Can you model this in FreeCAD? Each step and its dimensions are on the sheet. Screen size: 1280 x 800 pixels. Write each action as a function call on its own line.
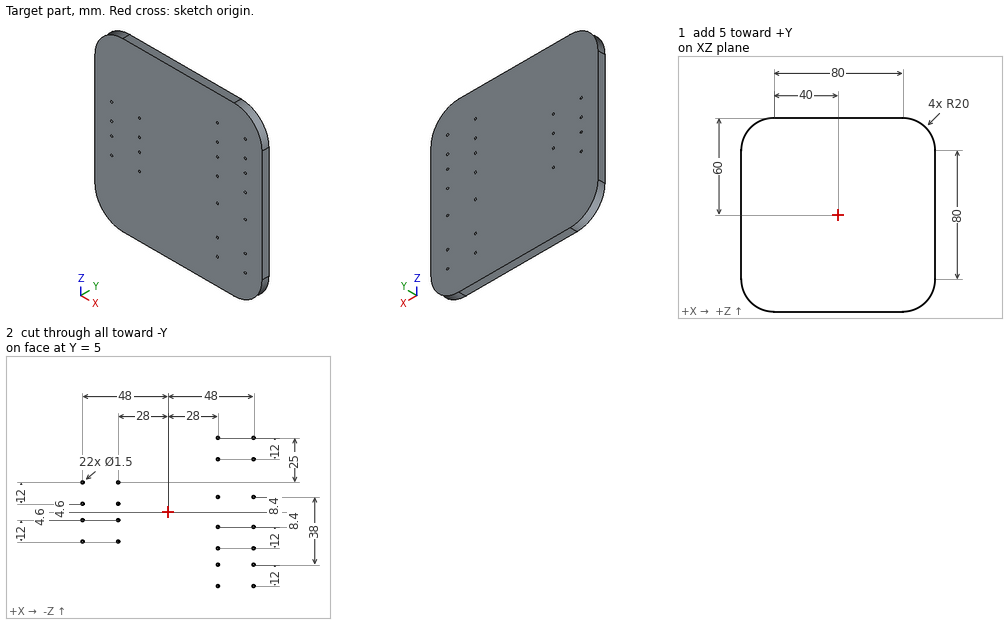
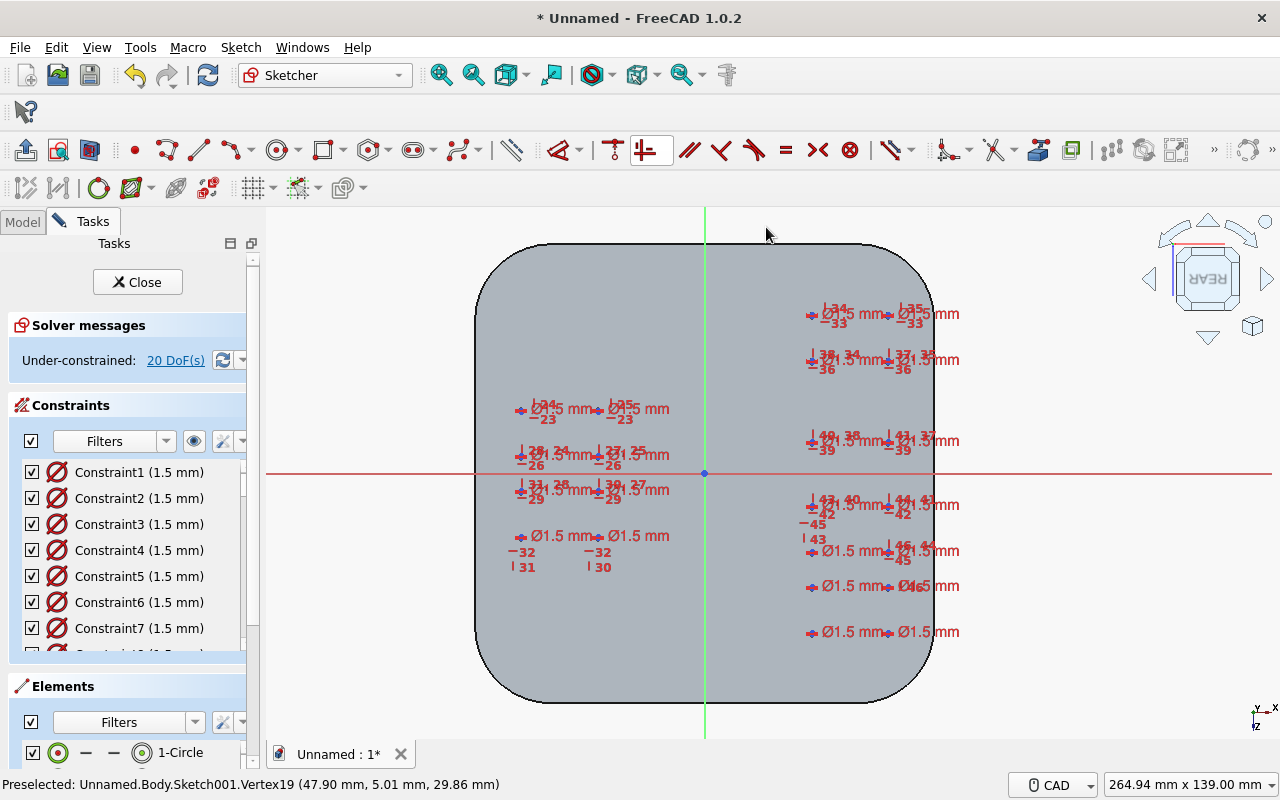
click(812, 553)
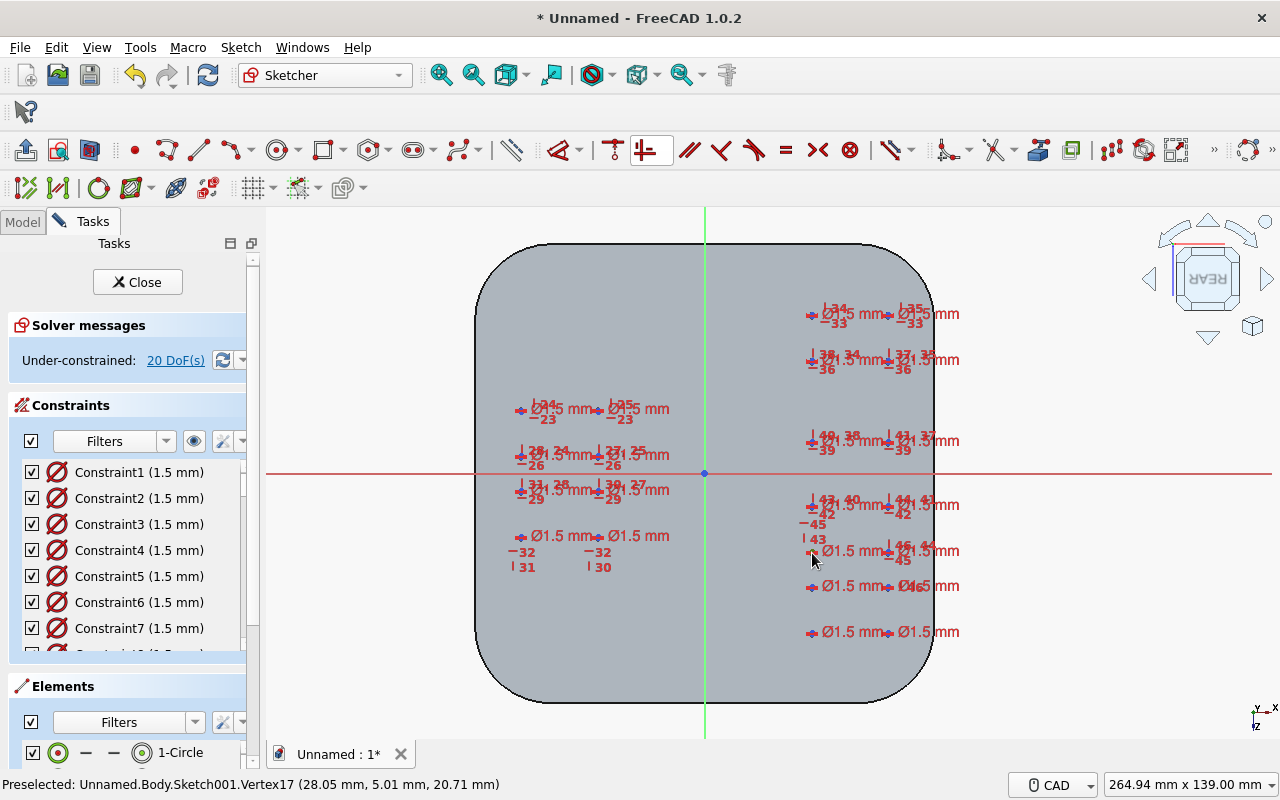
click(812, 588)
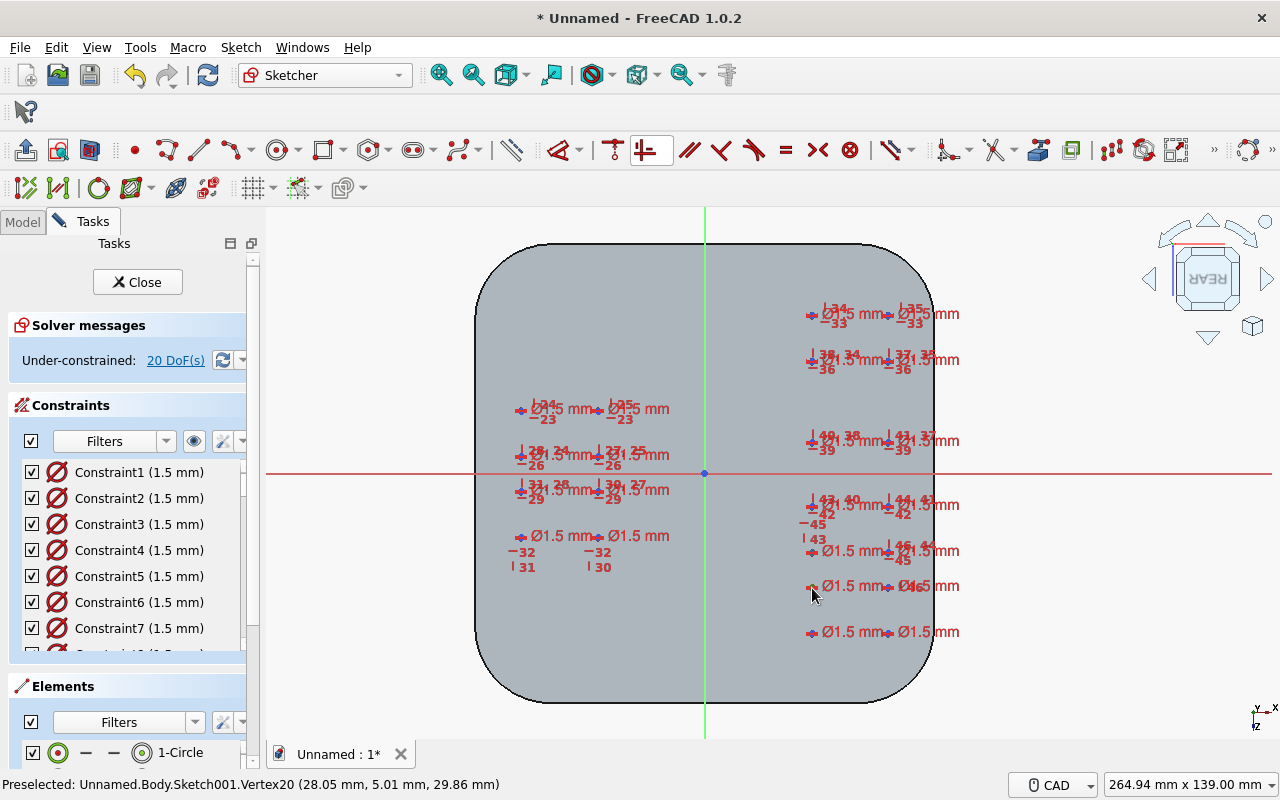
click(668, 150)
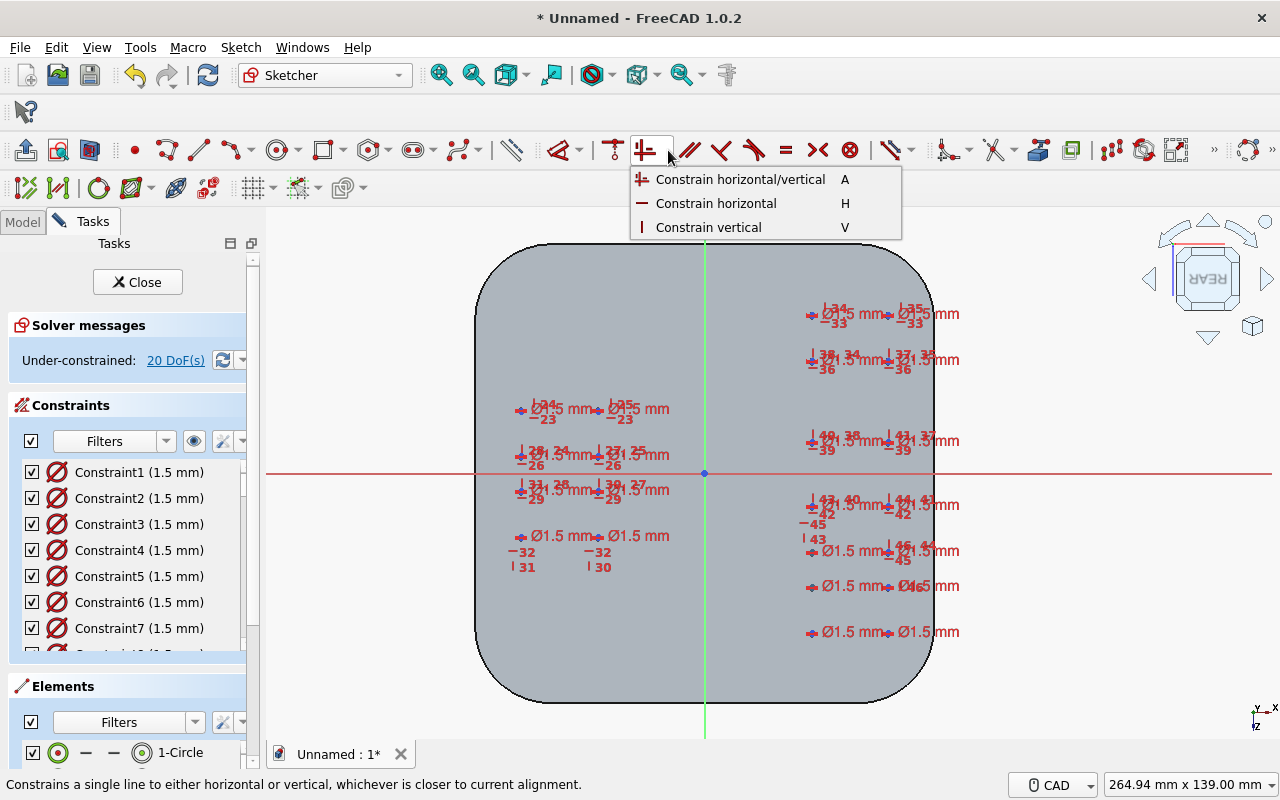
click(766, 227)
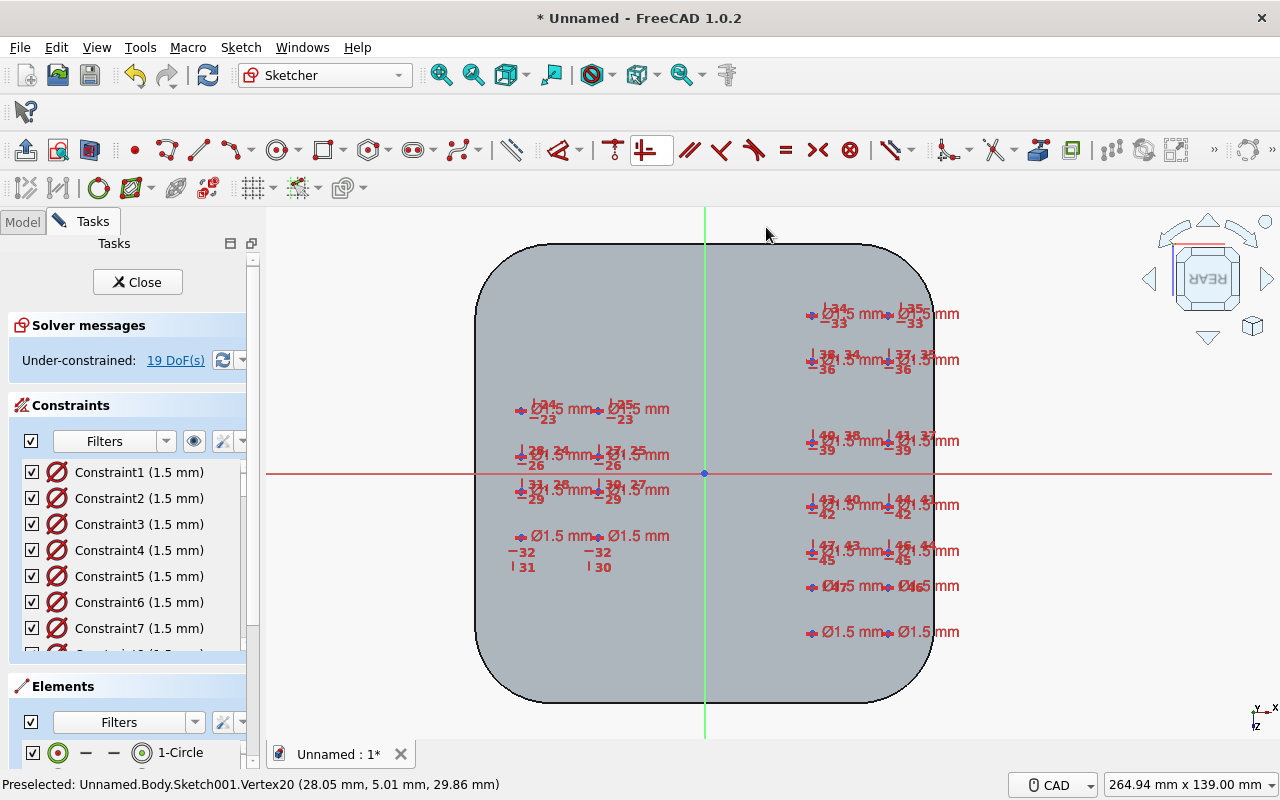
click(888, 588)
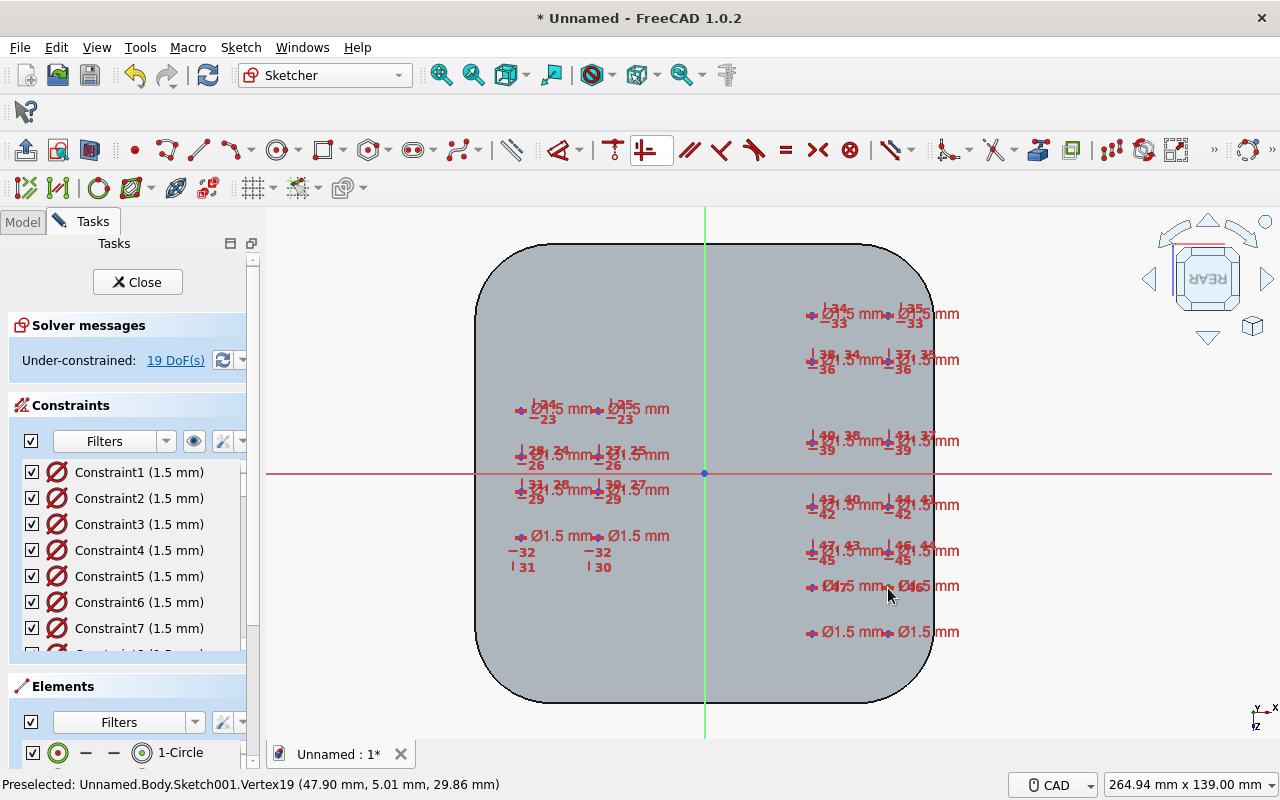
click(812, 588)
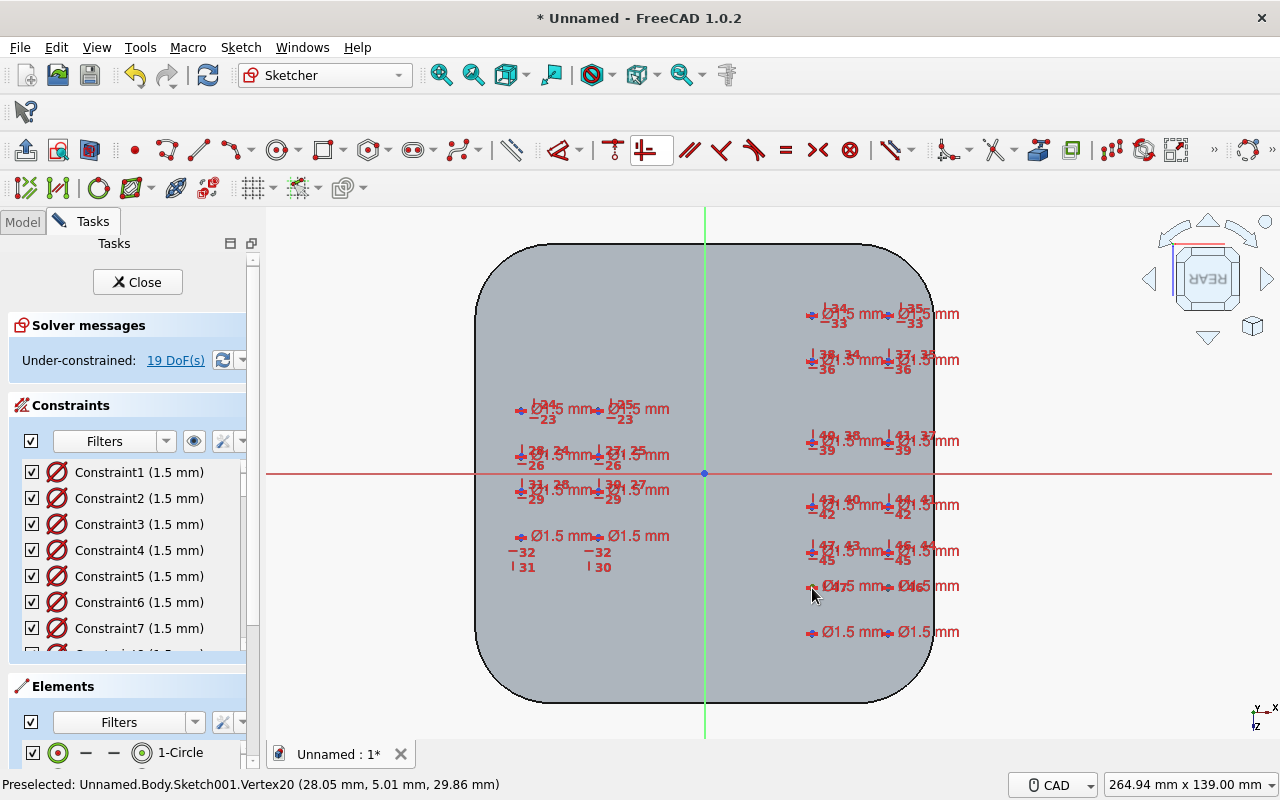
click(668, 150)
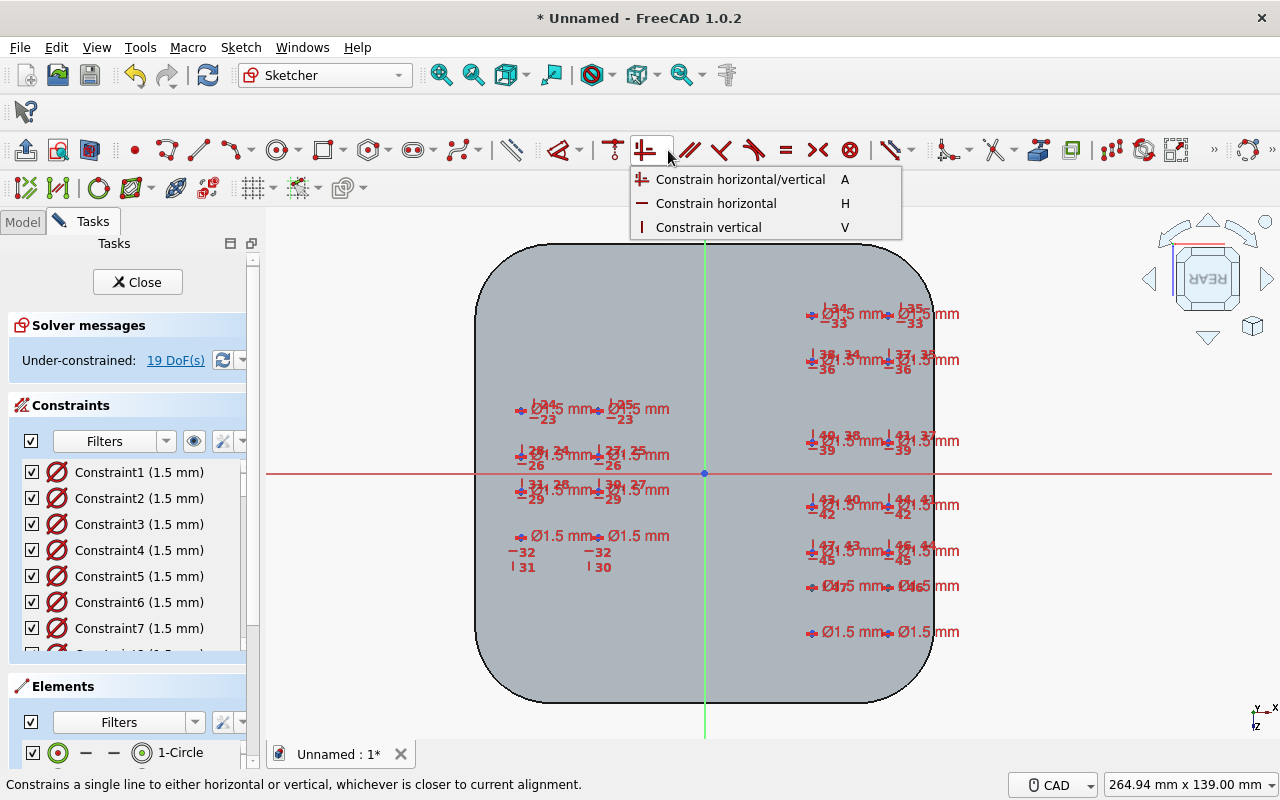
click(766, 203)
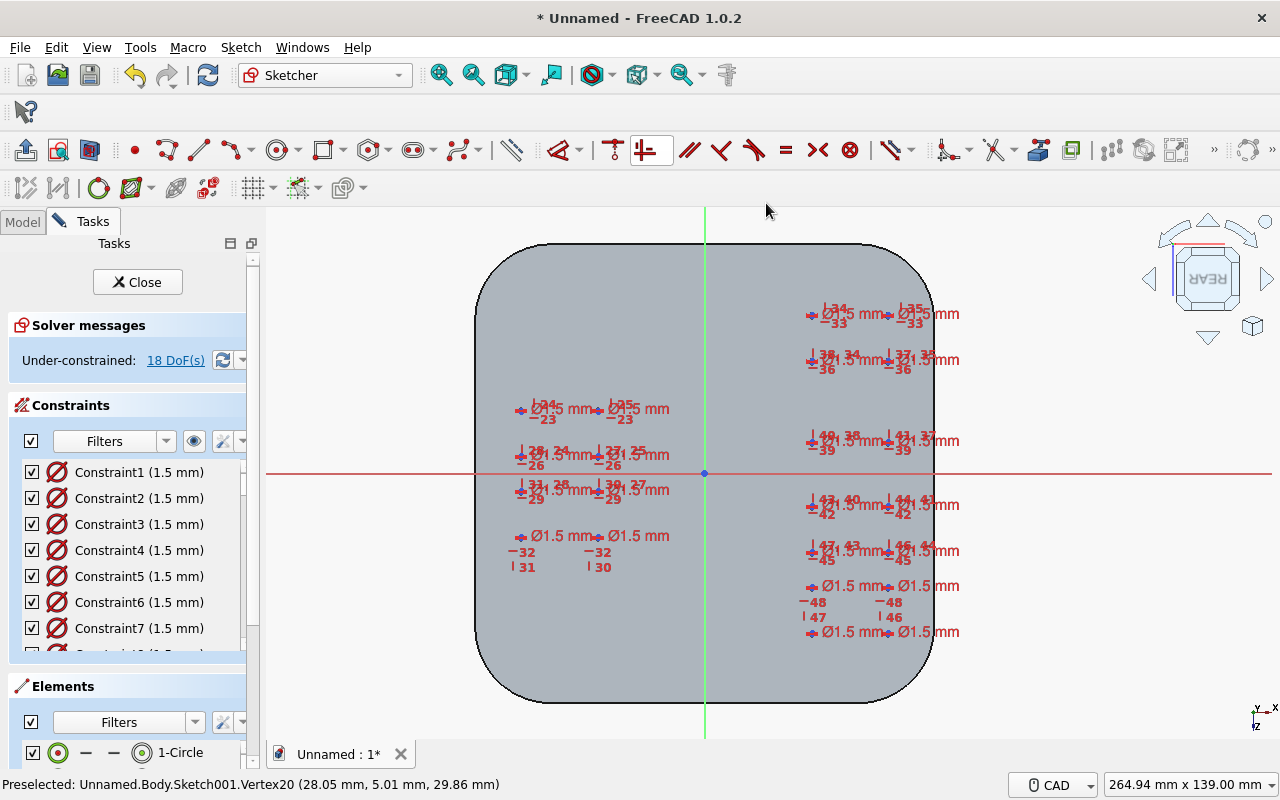
click(888, 588)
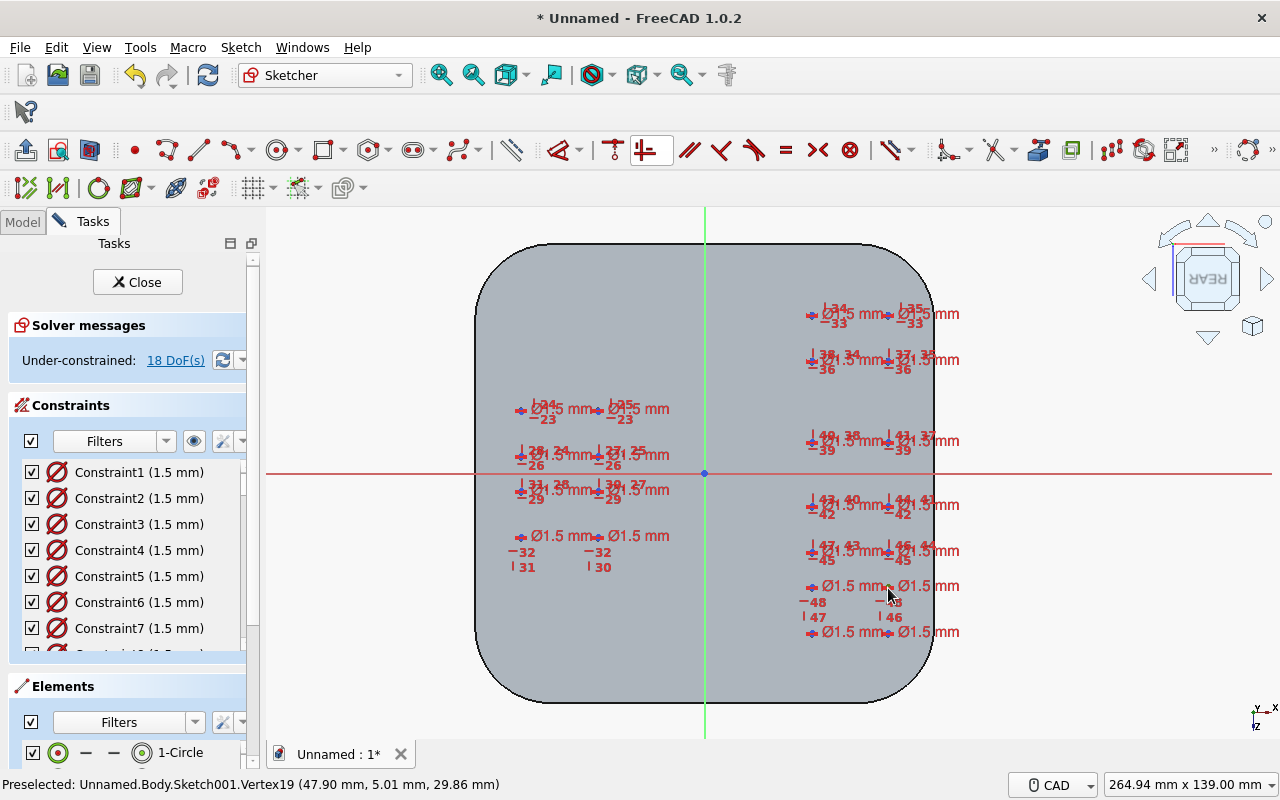
click(888, 634)